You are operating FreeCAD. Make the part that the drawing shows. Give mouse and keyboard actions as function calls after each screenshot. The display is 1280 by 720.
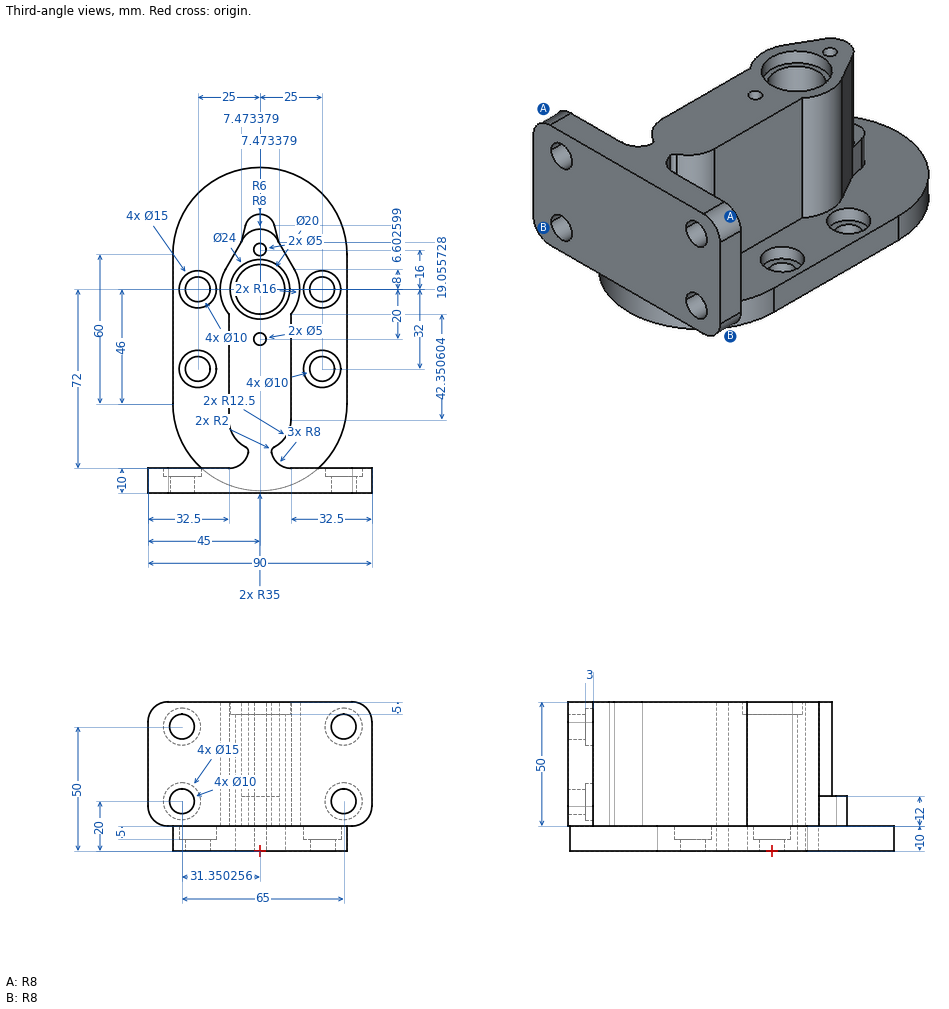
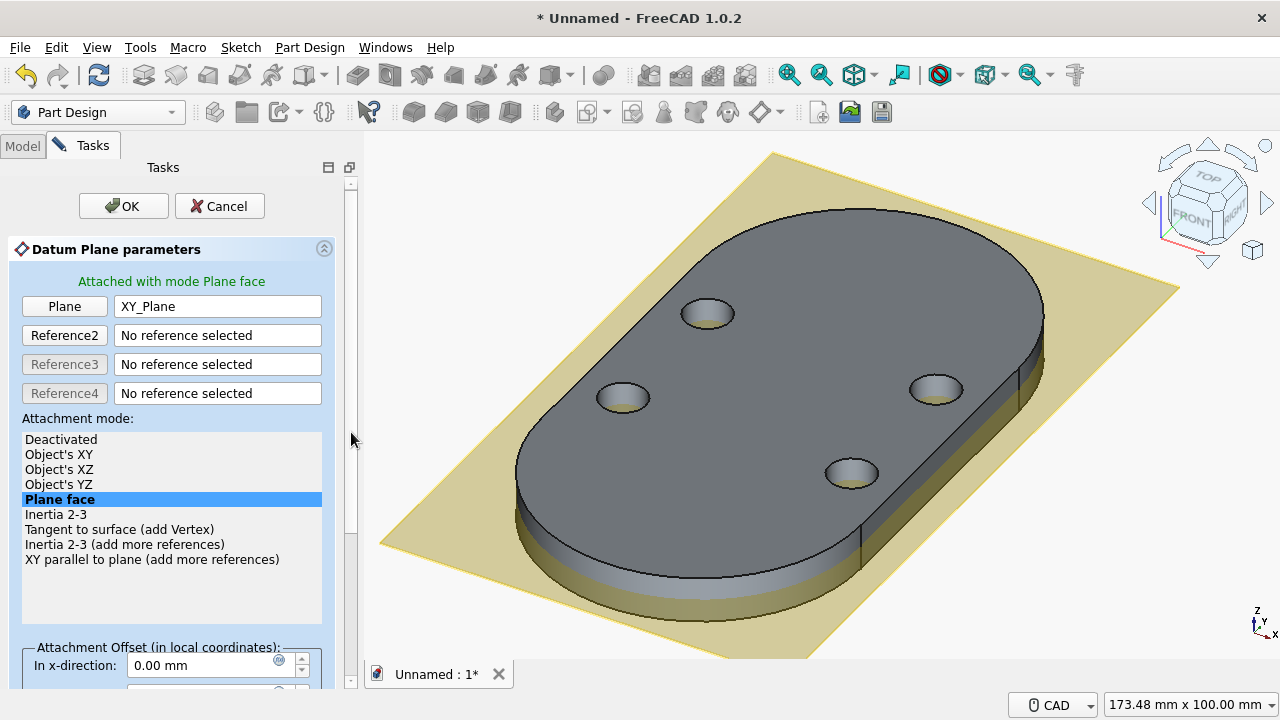
click(124, 206)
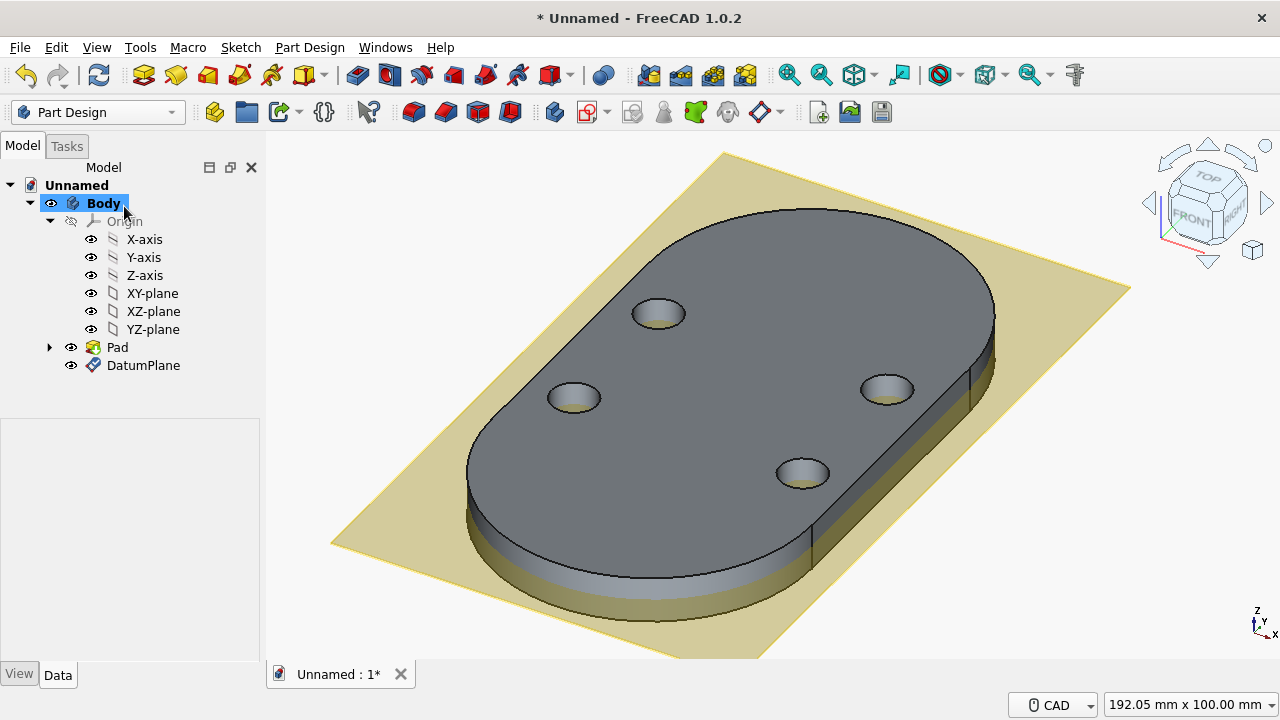
click(116, 365)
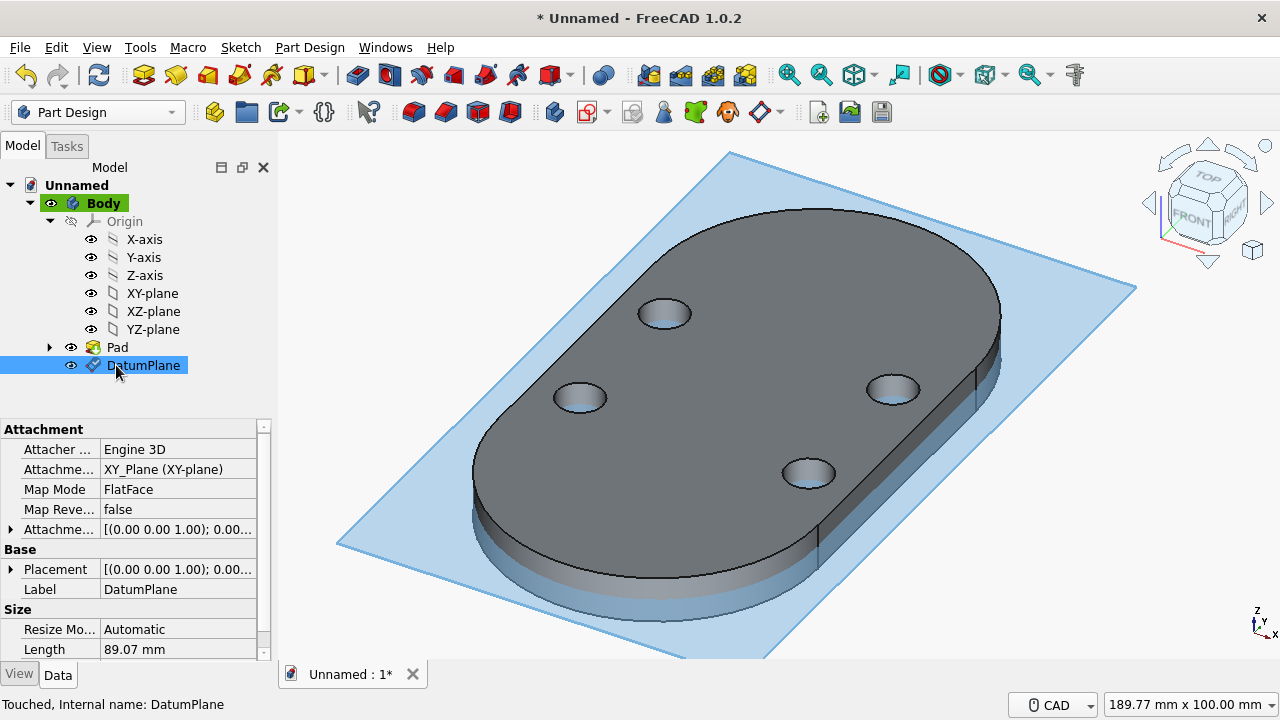
click(588, 112)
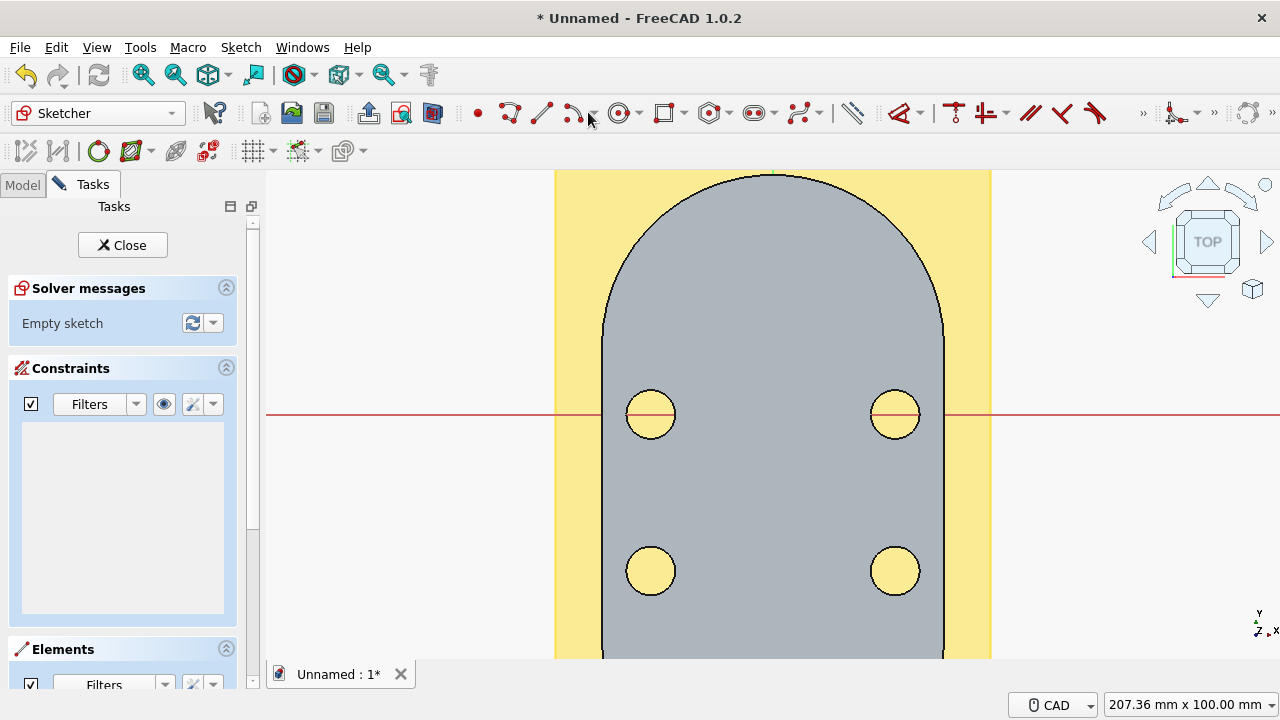
click(434, 114)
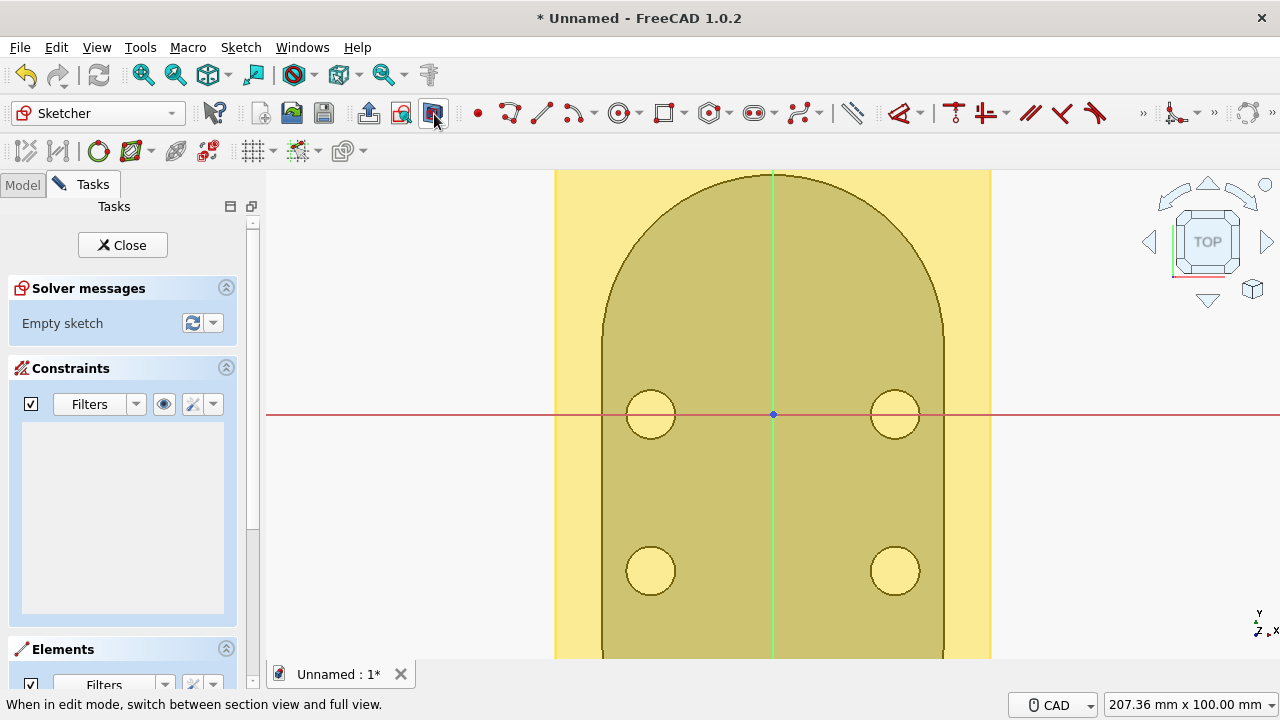
scroll(1082, 631, up, 1)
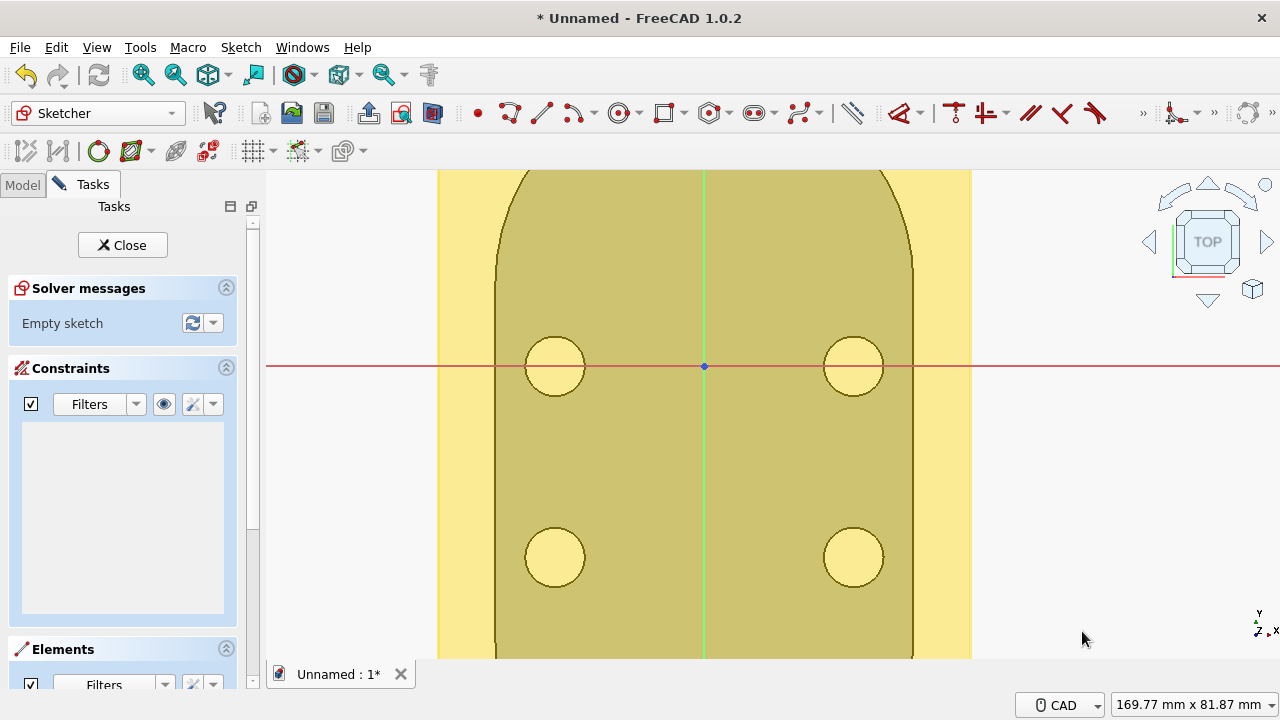
click(620, 114)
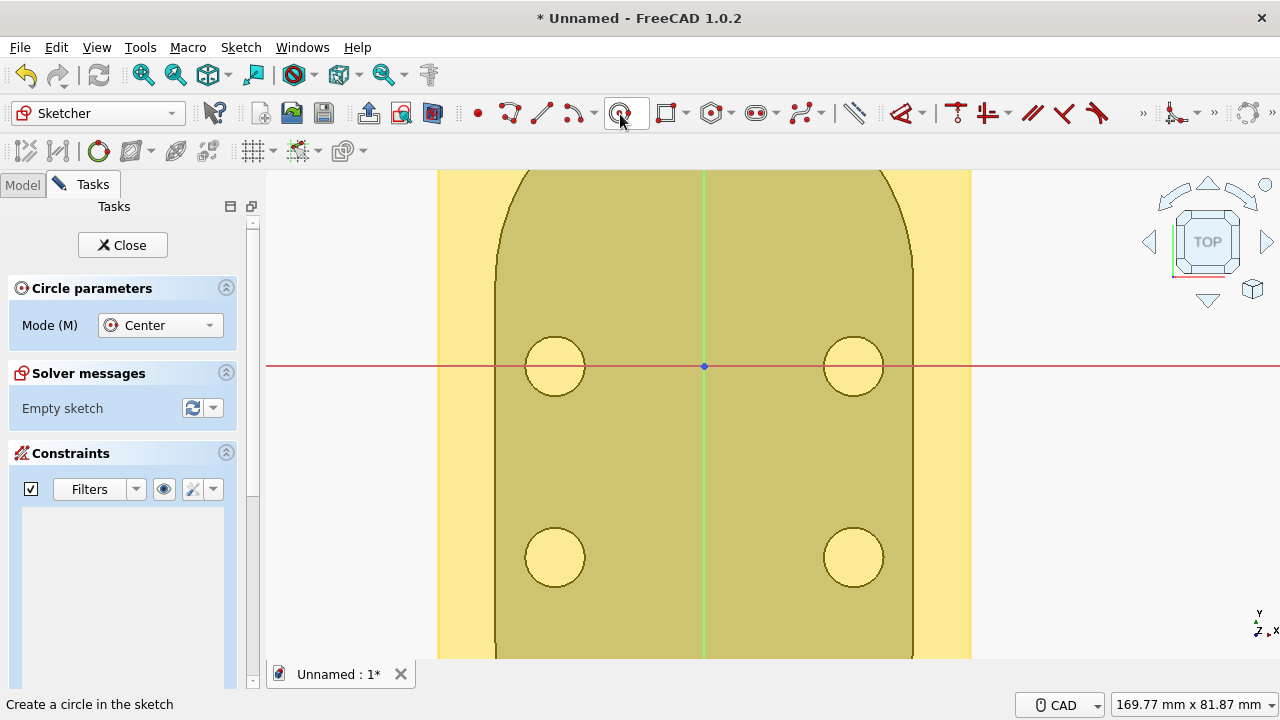
click(555, 366)
click(587, 335)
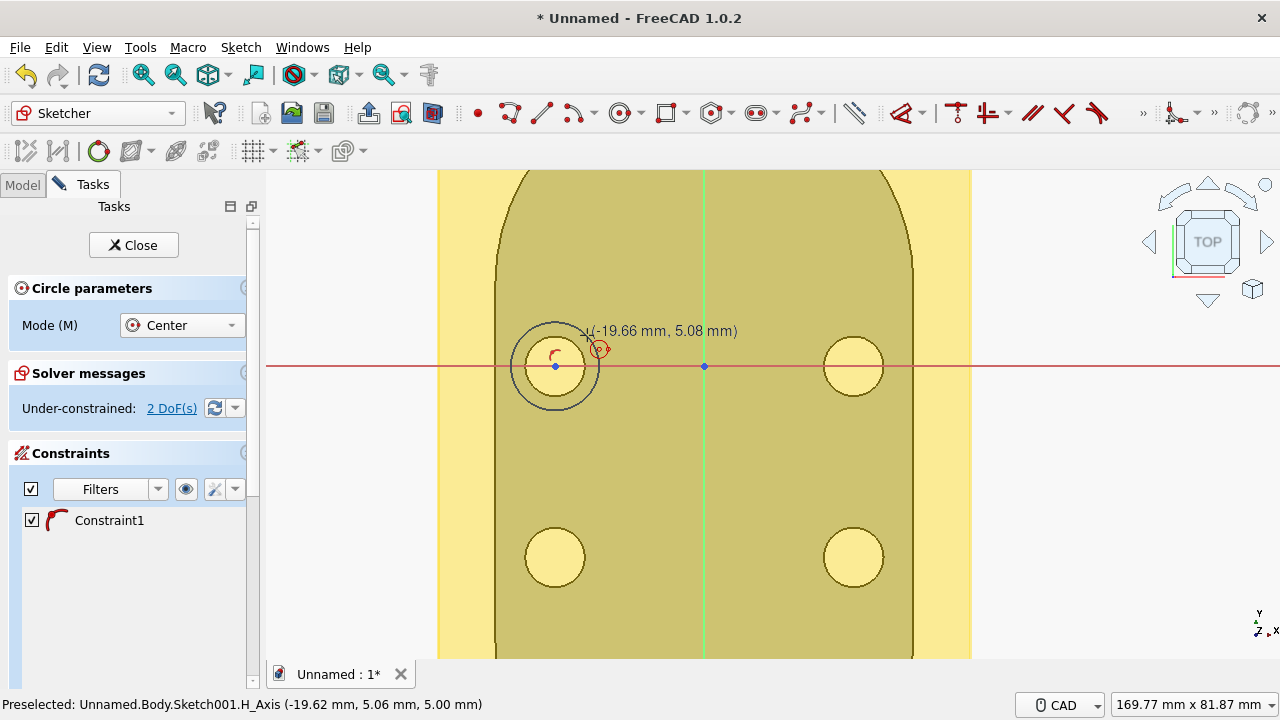
click(854, 366)
click(885, 335)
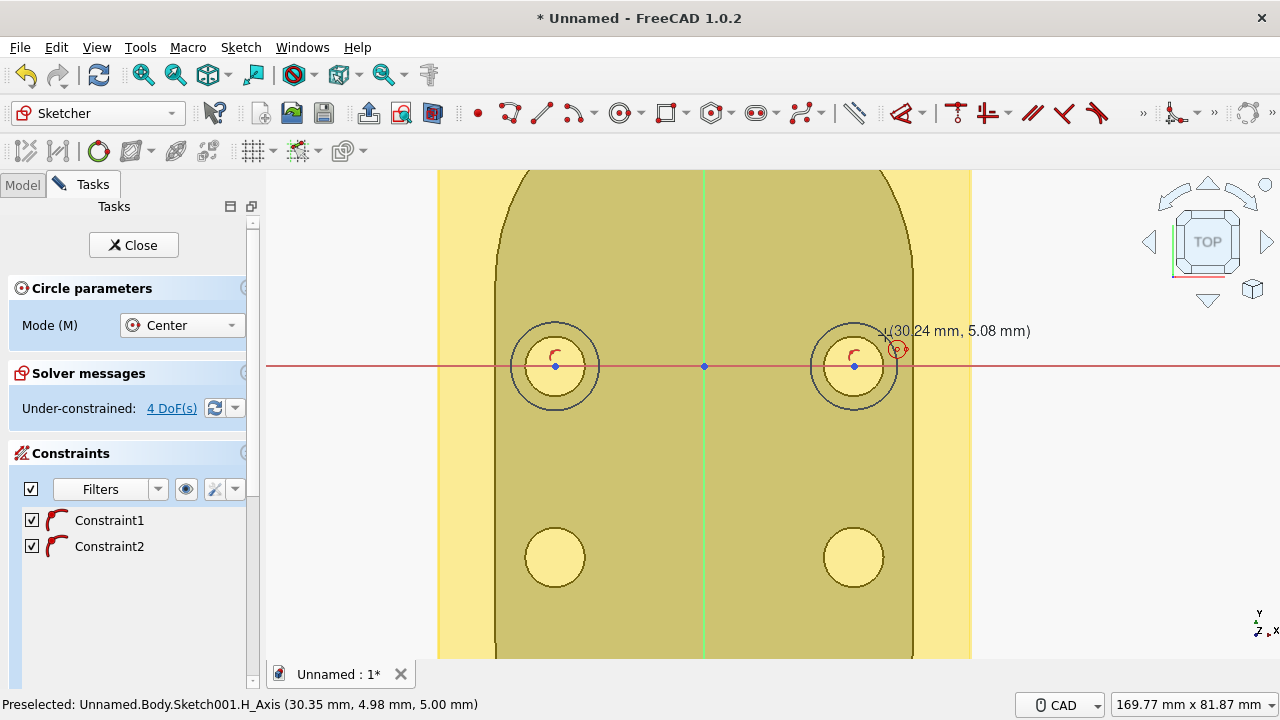
click(854, 557)
click(885, 526)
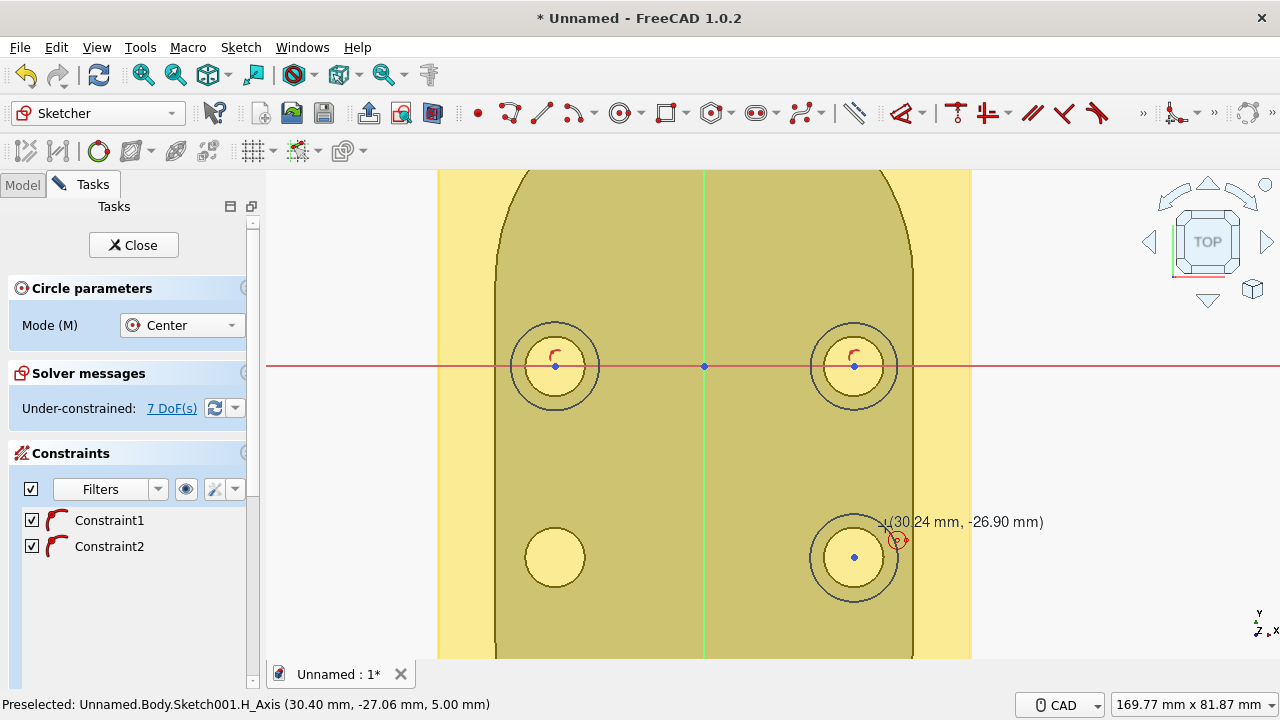
click(555, 557)
click(587, 526)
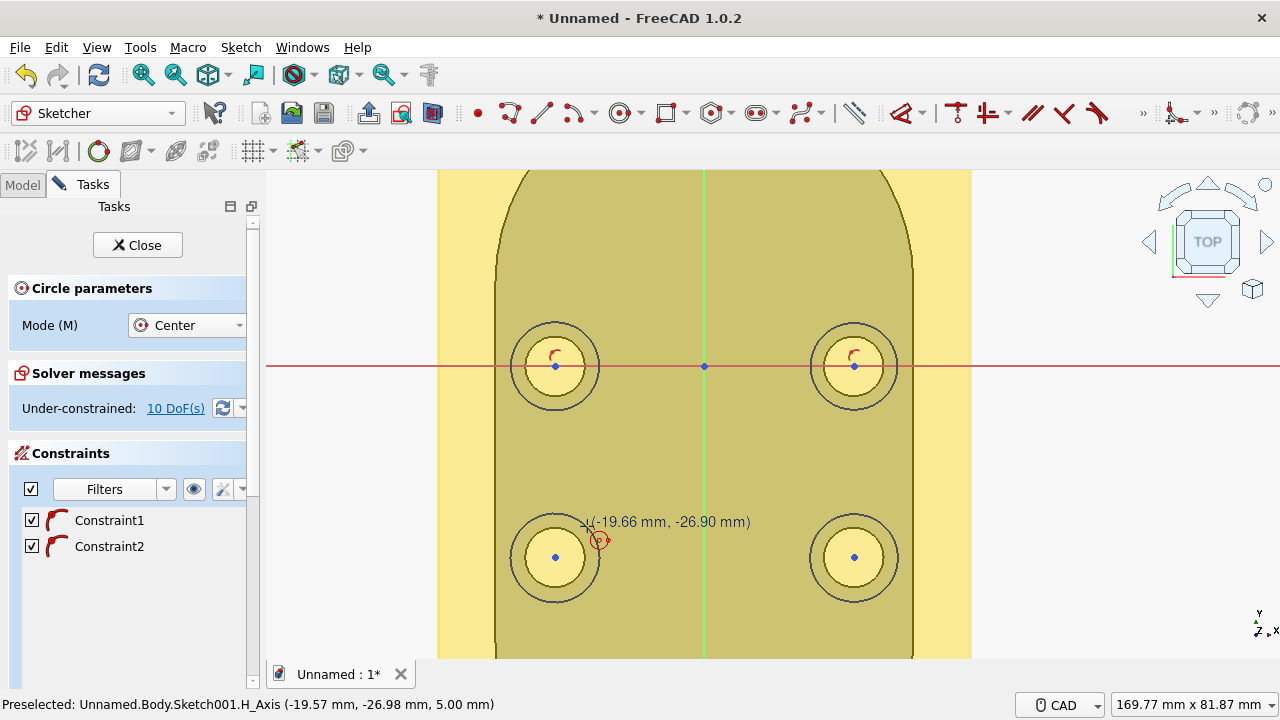
click(555, 366)
click(576, 345)